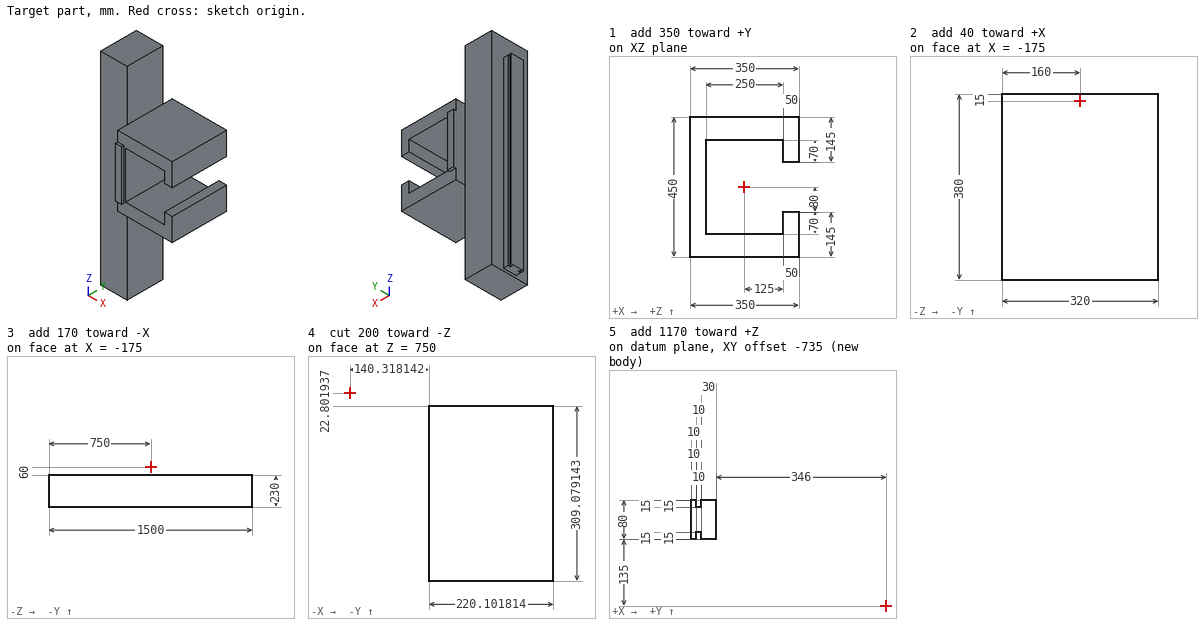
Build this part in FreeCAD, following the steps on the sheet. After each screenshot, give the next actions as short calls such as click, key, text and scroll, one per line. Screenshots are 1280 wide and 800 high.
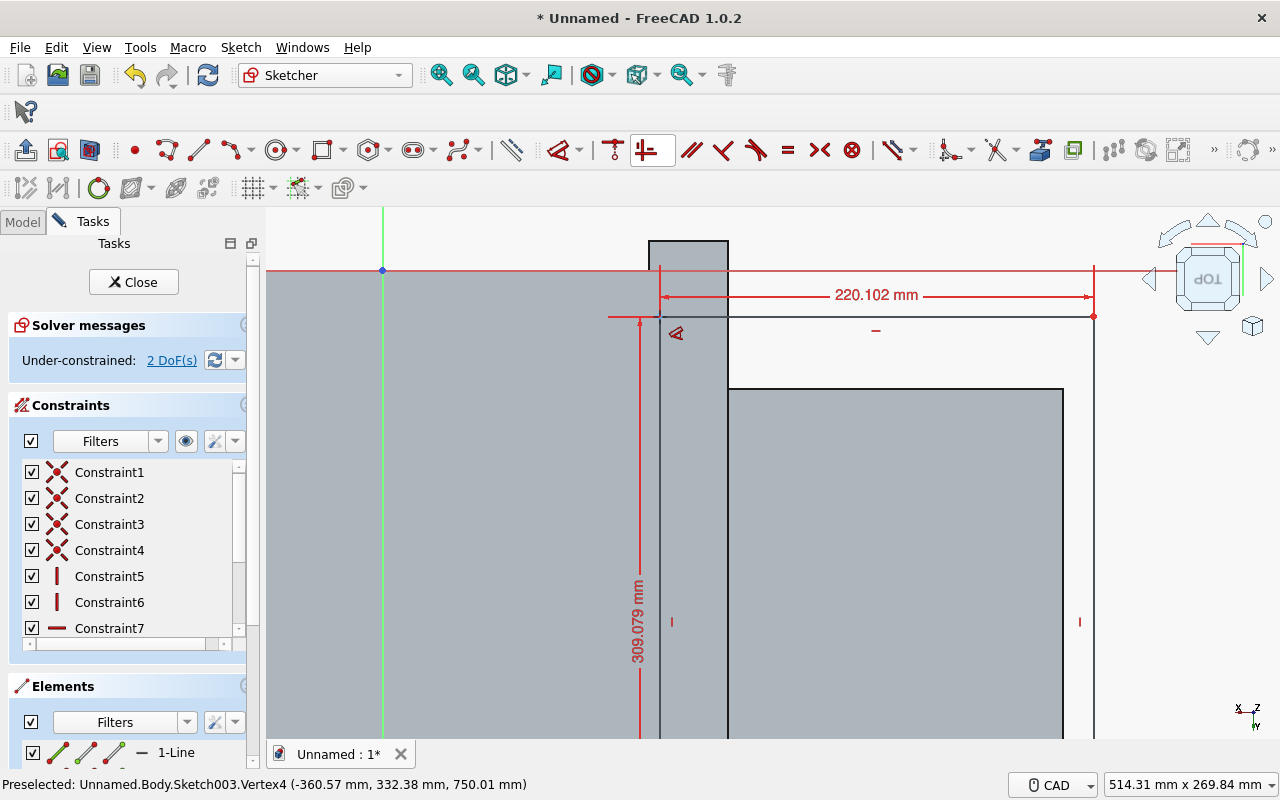
click(660, 317)
click(349, 294)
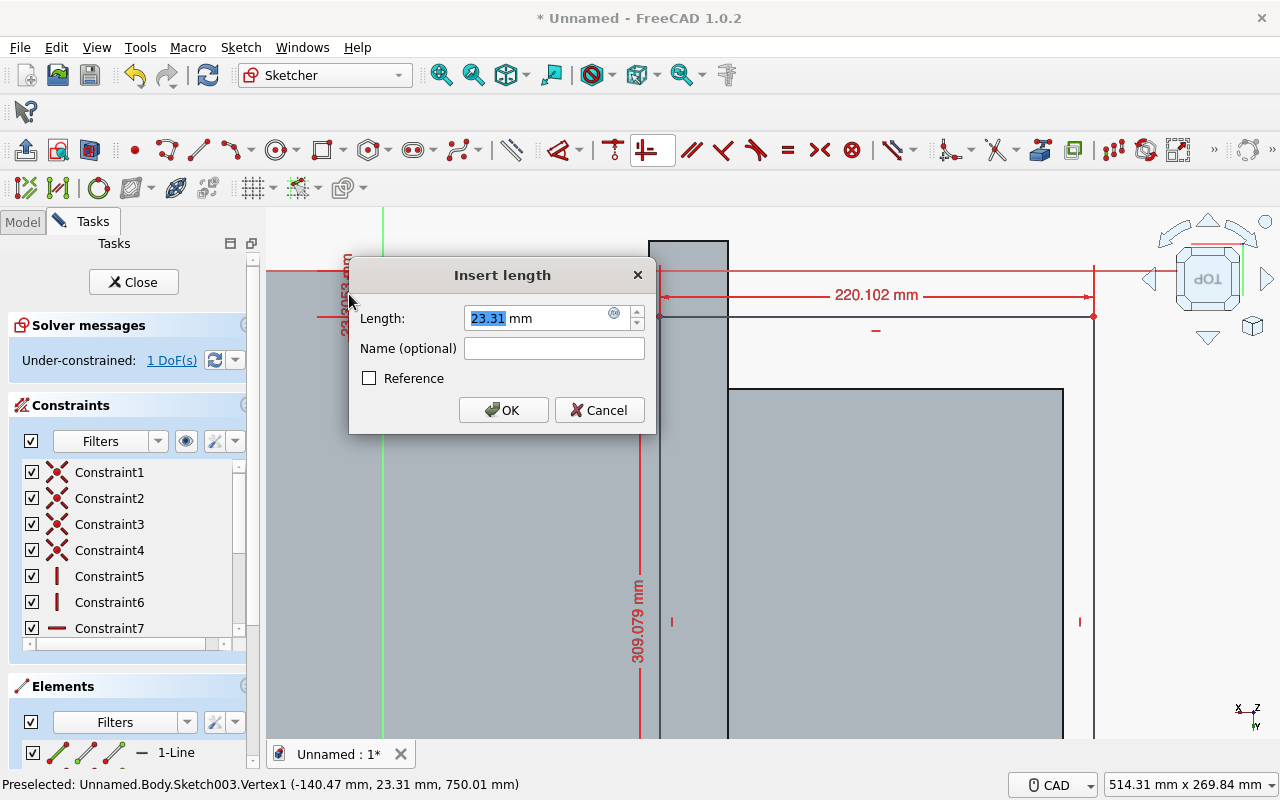
text(22.801937)
key(Return)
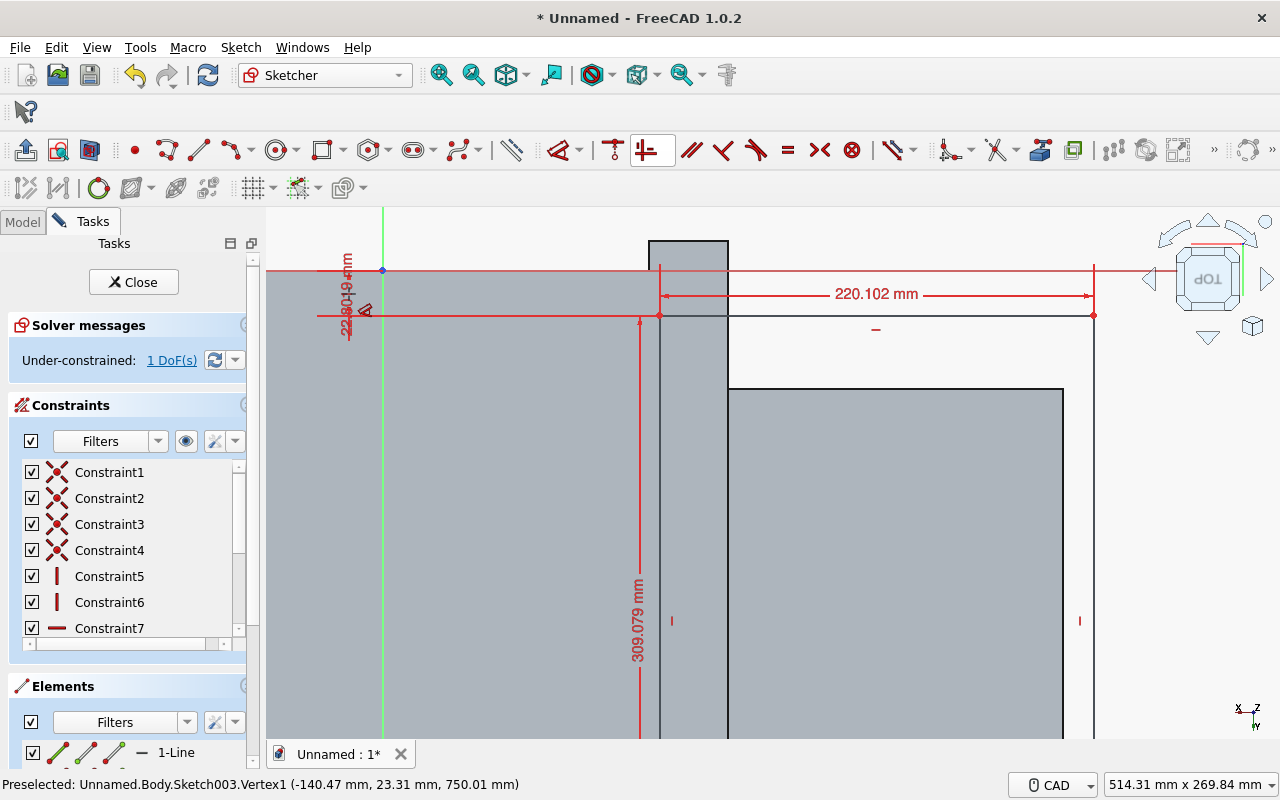
click(660, 316)
click(521, 237)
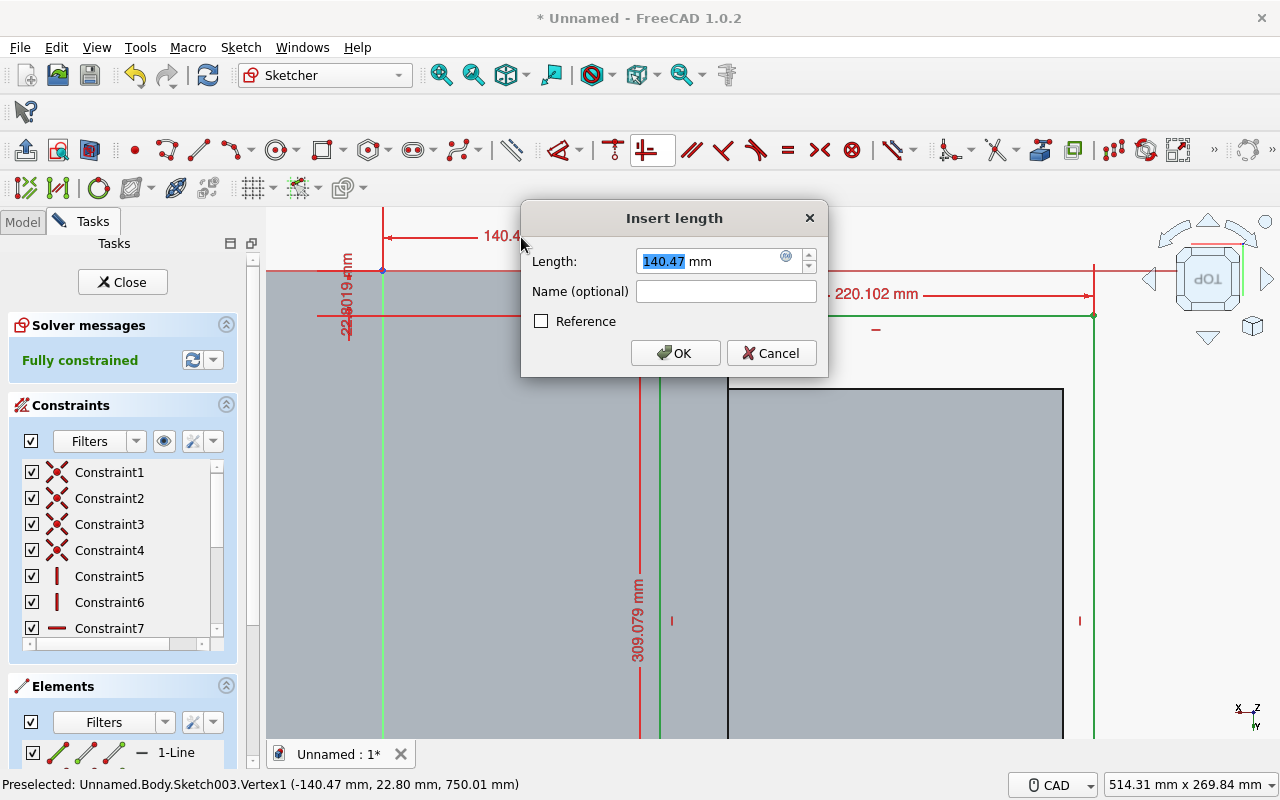
text(140.318142)
key(Return)
key(Escape)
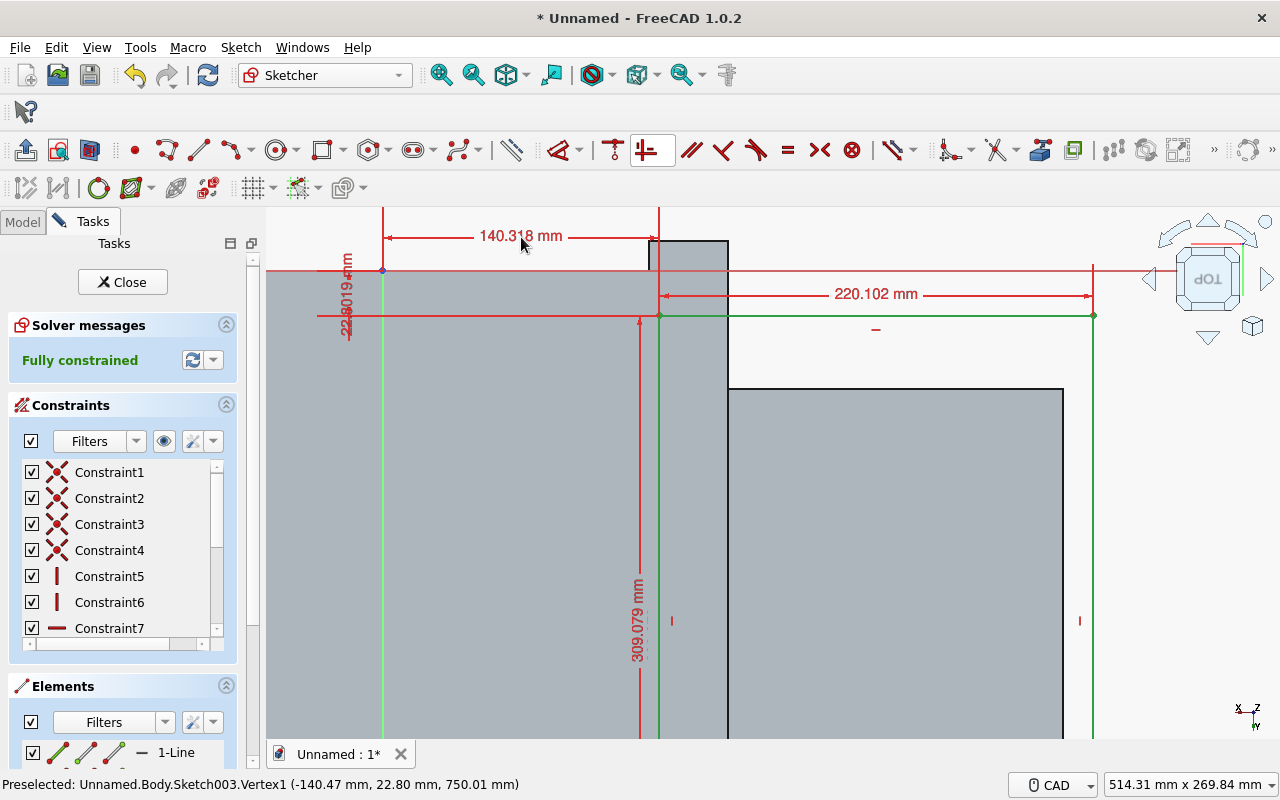
click(123, 282)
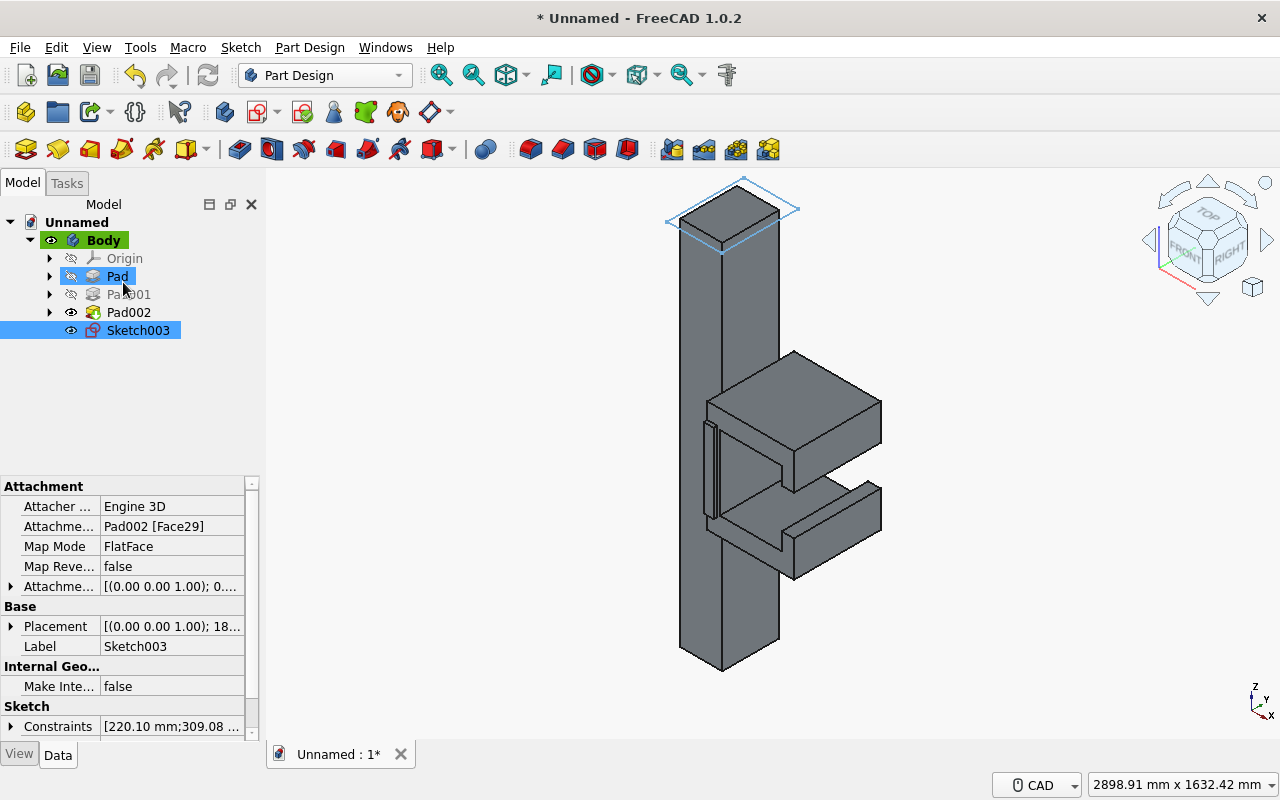
click(240, 150)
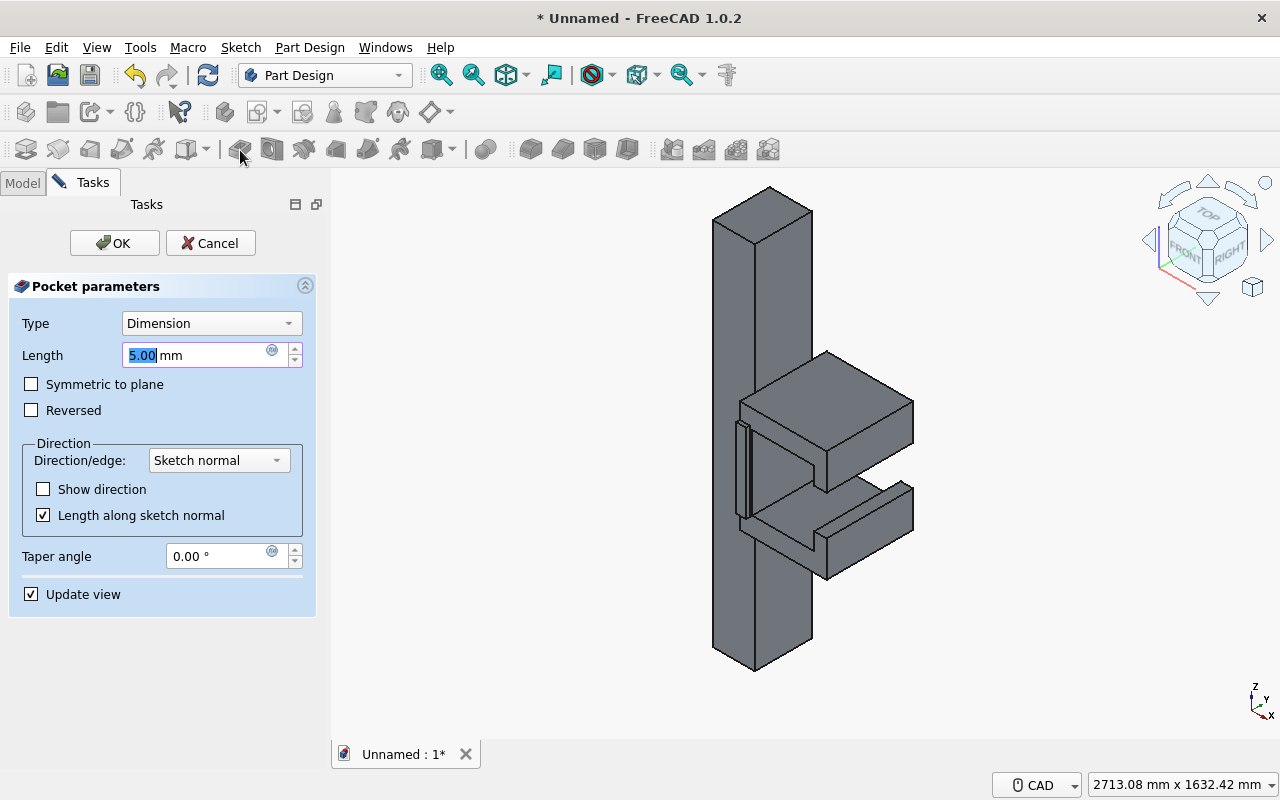
text(200)
key(Tab)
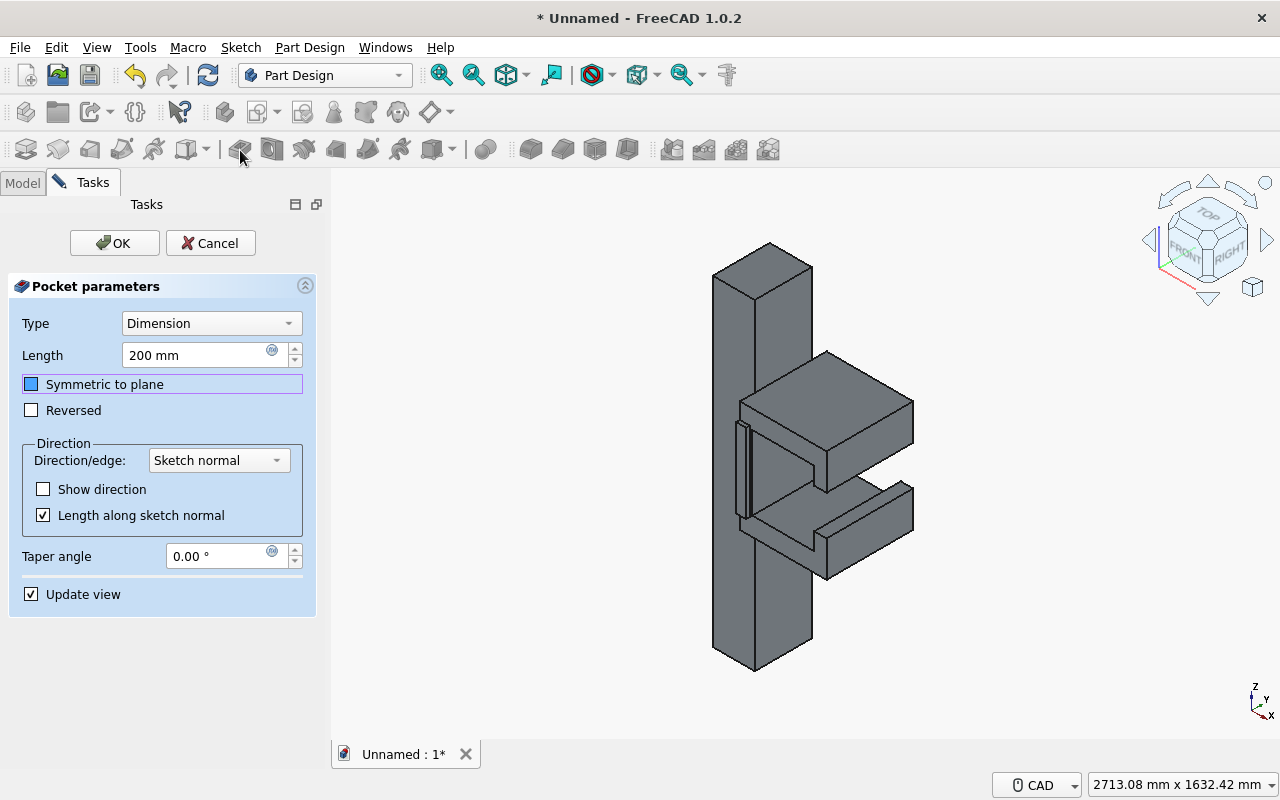
click(115, 243)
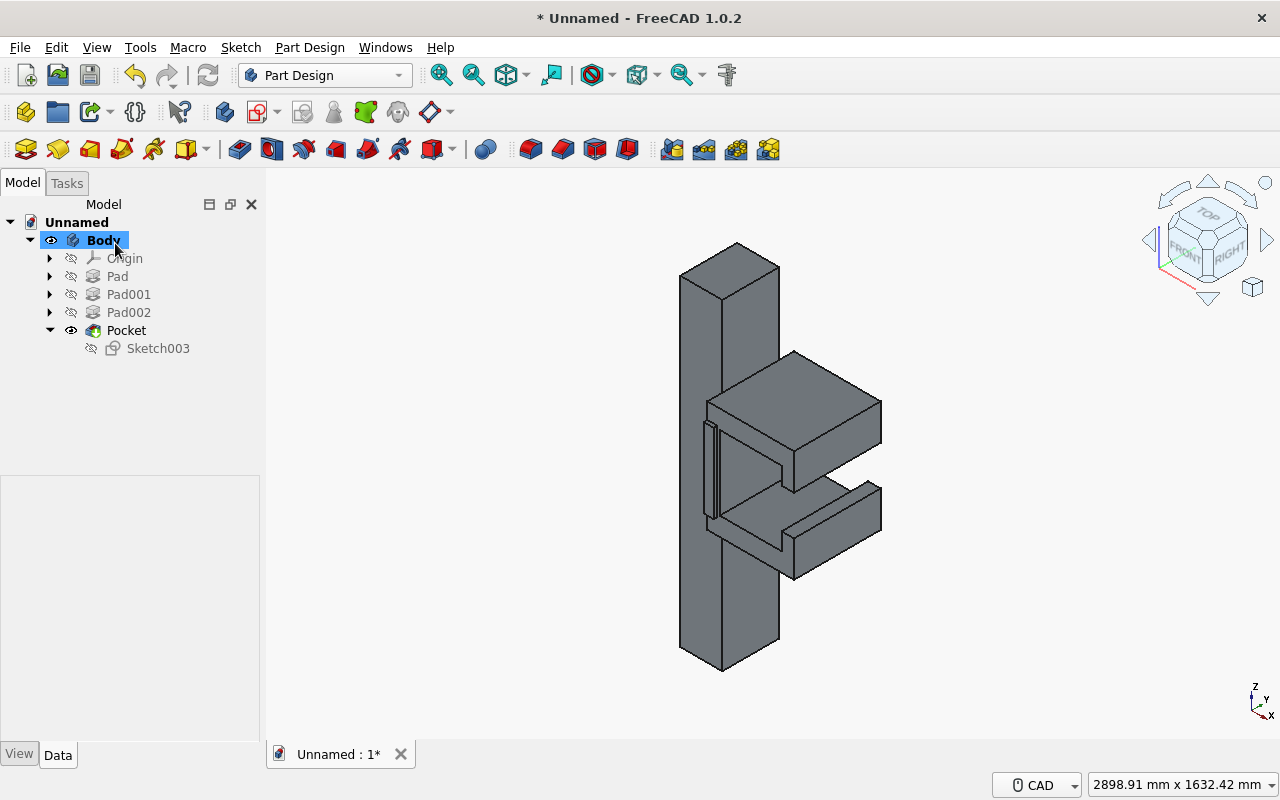
click(226, 112)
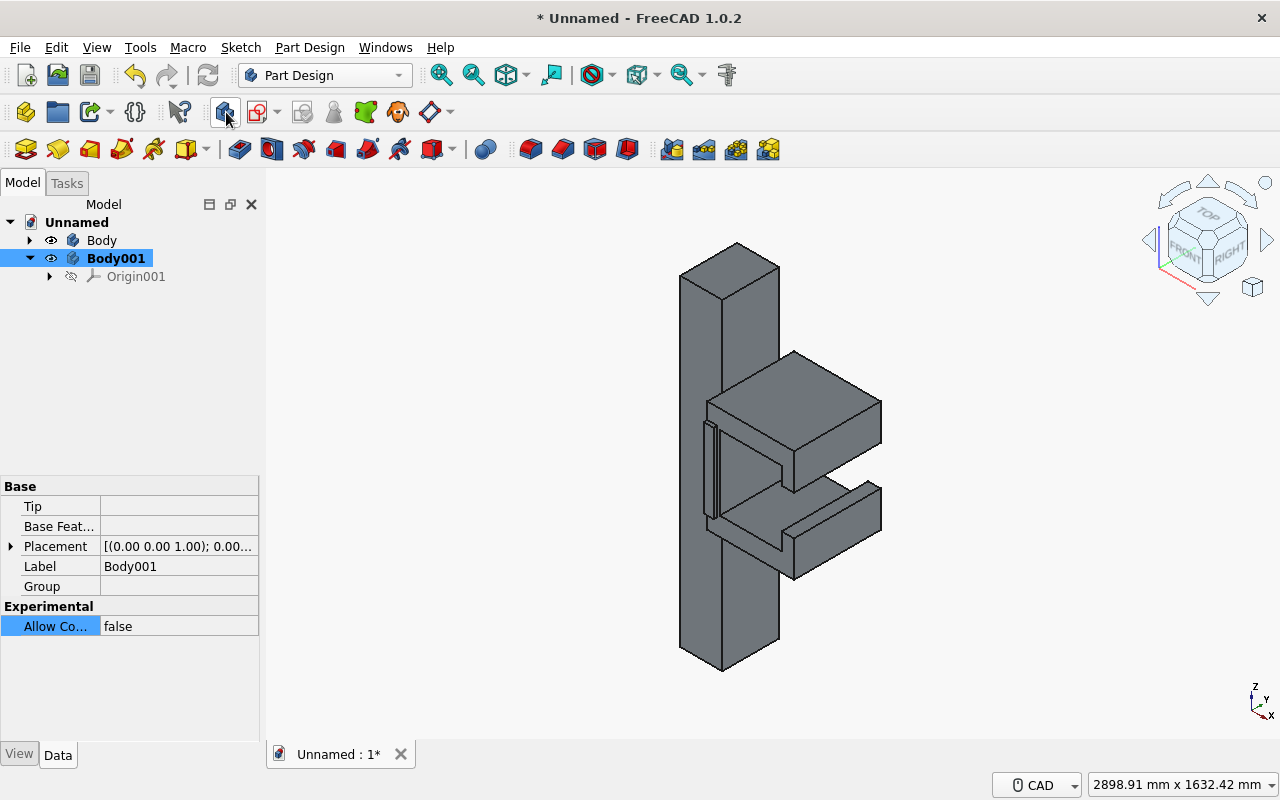
click(50, 276)